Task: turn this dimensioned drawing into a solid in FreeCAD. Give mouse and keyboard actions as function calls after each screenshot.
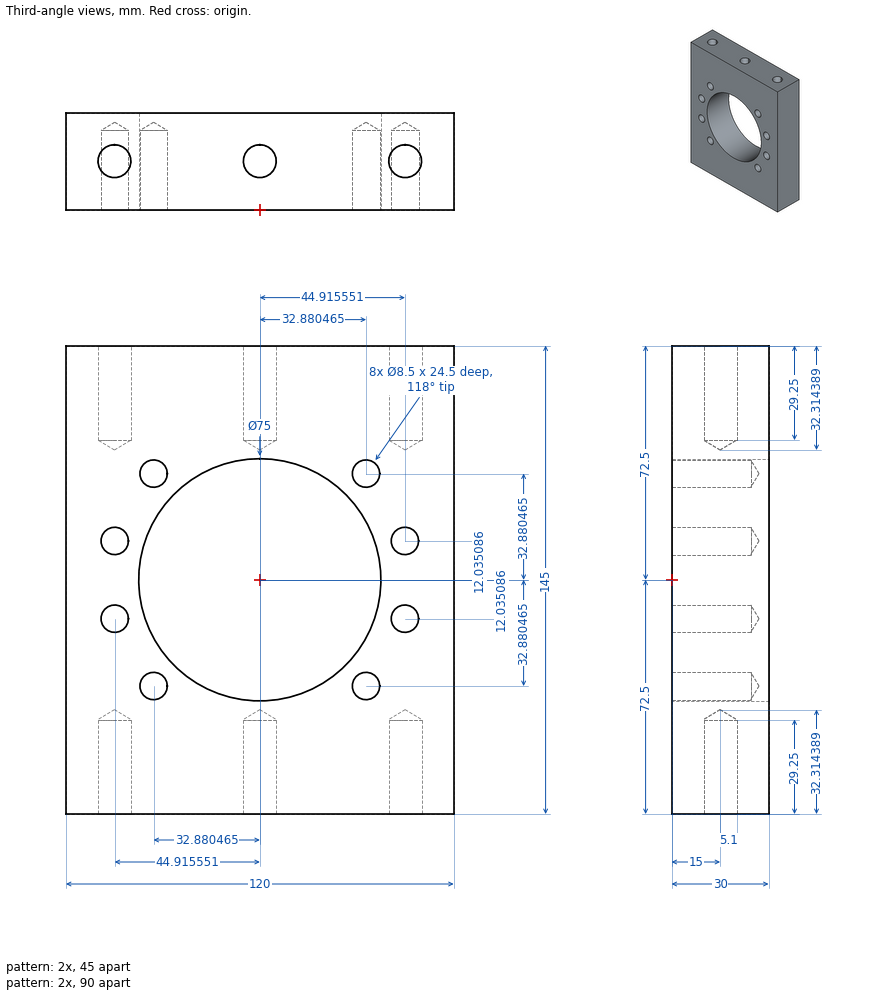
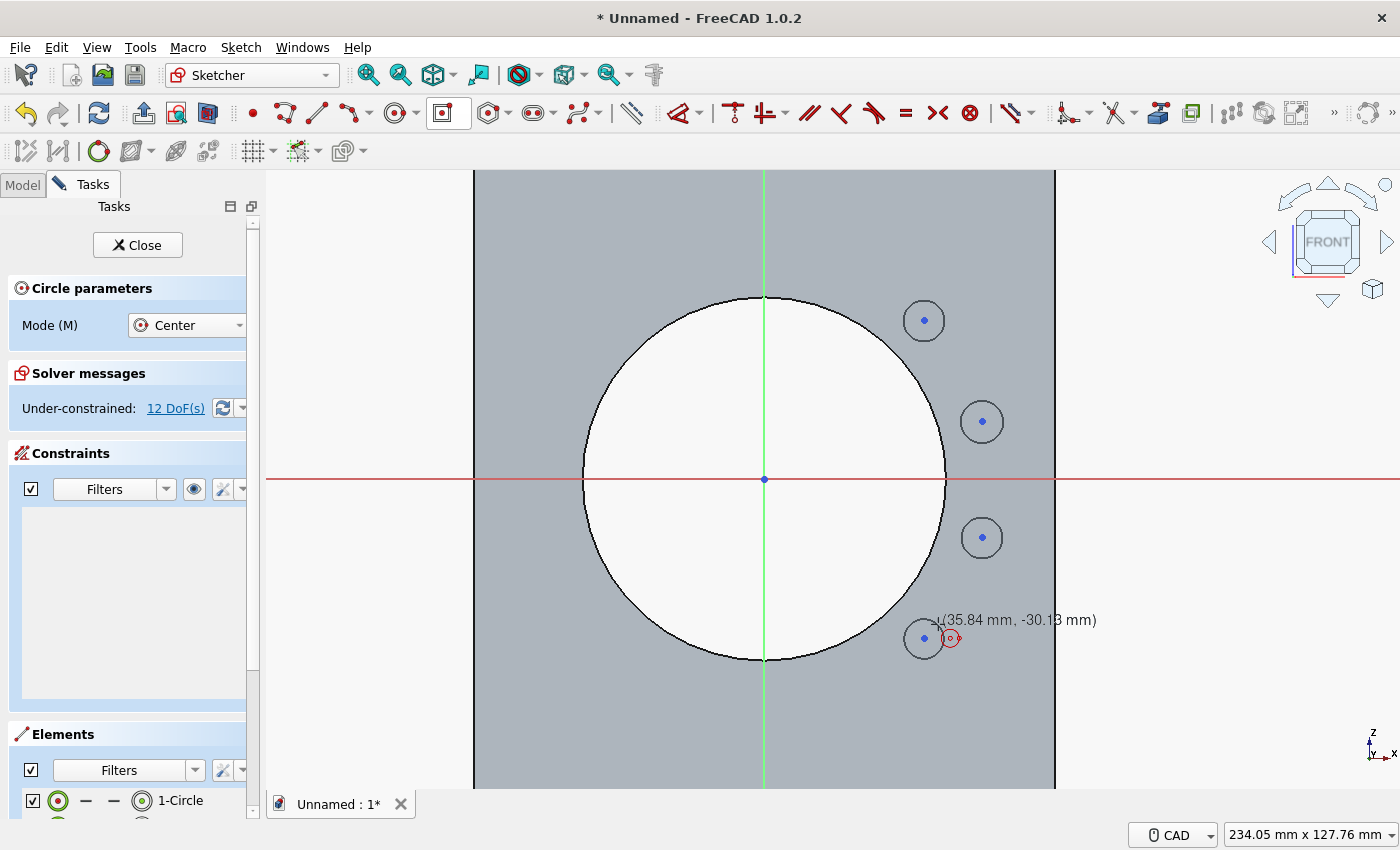
click(605, 638)
click(620, 624)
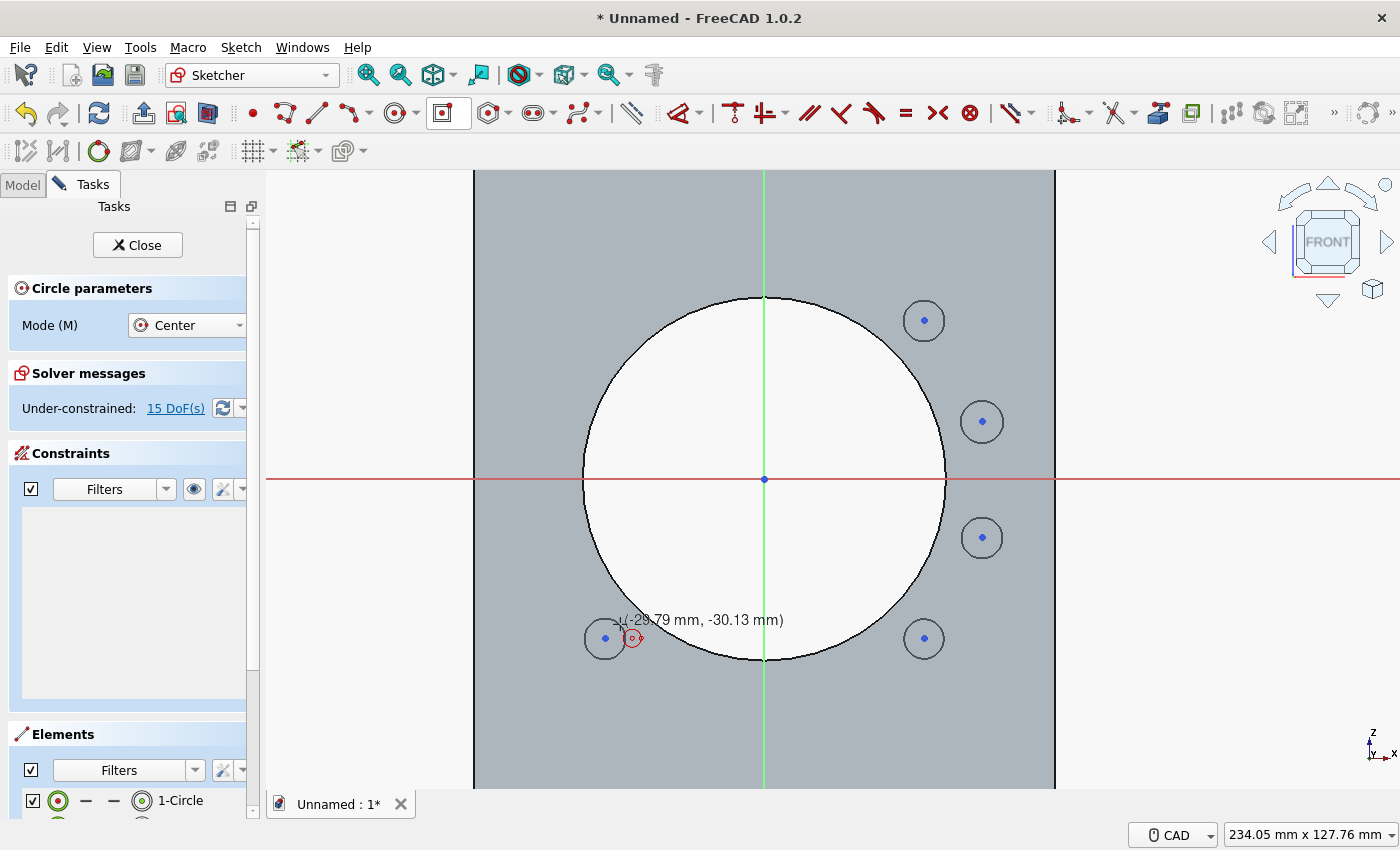
click(547, 537)
click(561, 523)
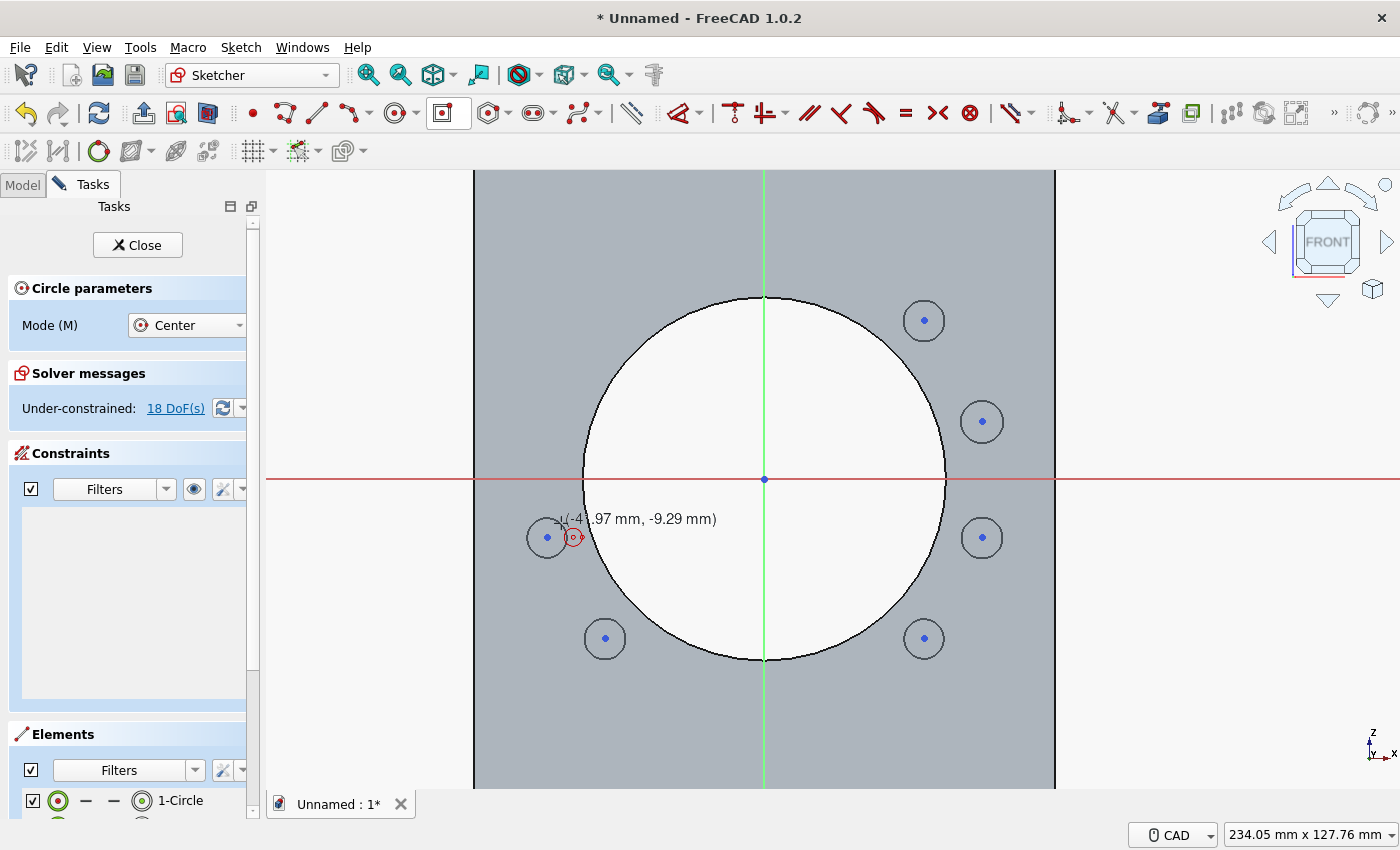
click(547, 421)
click(561, 406)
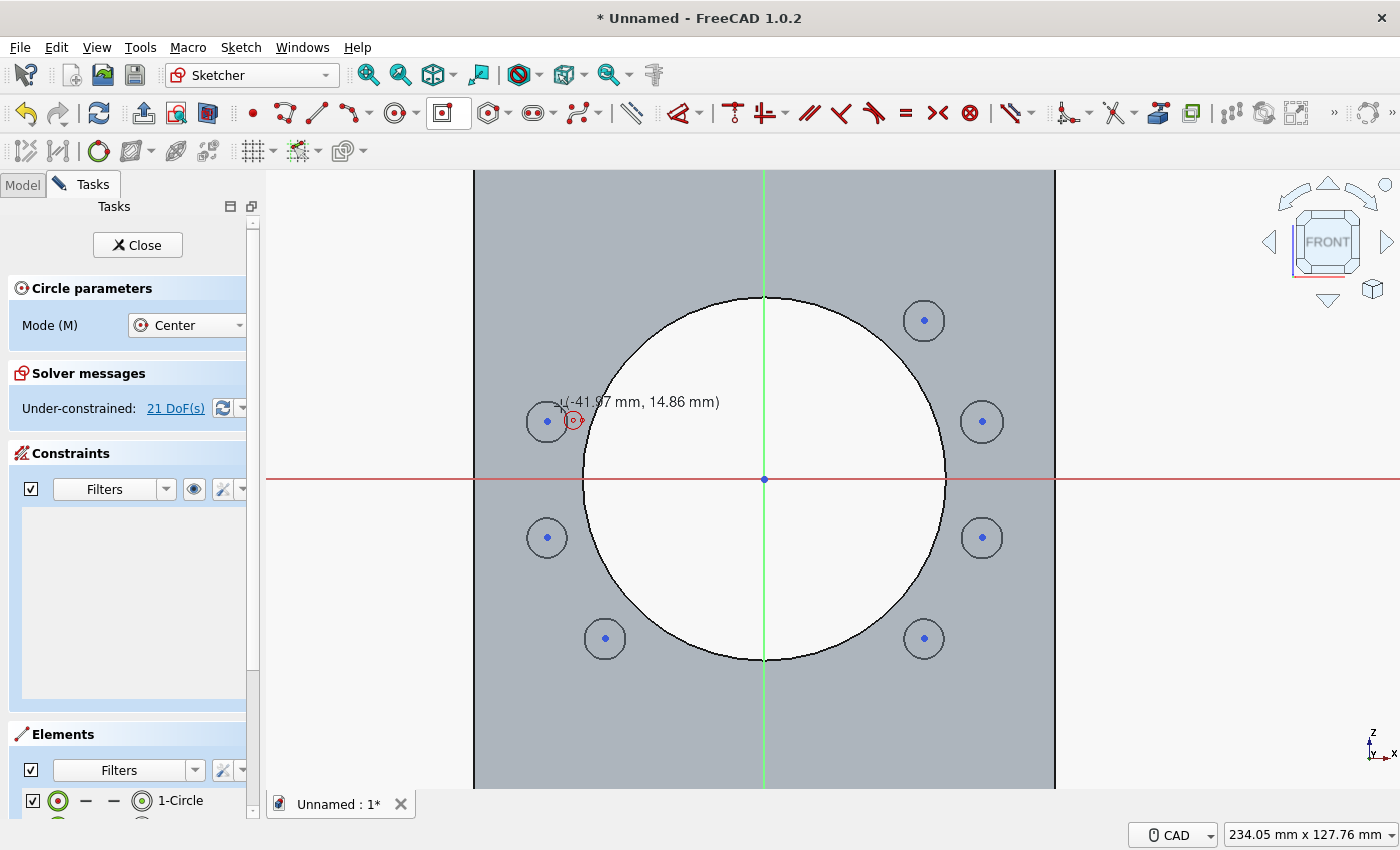
click(605, 320)
click(620, 305)
key(Escape)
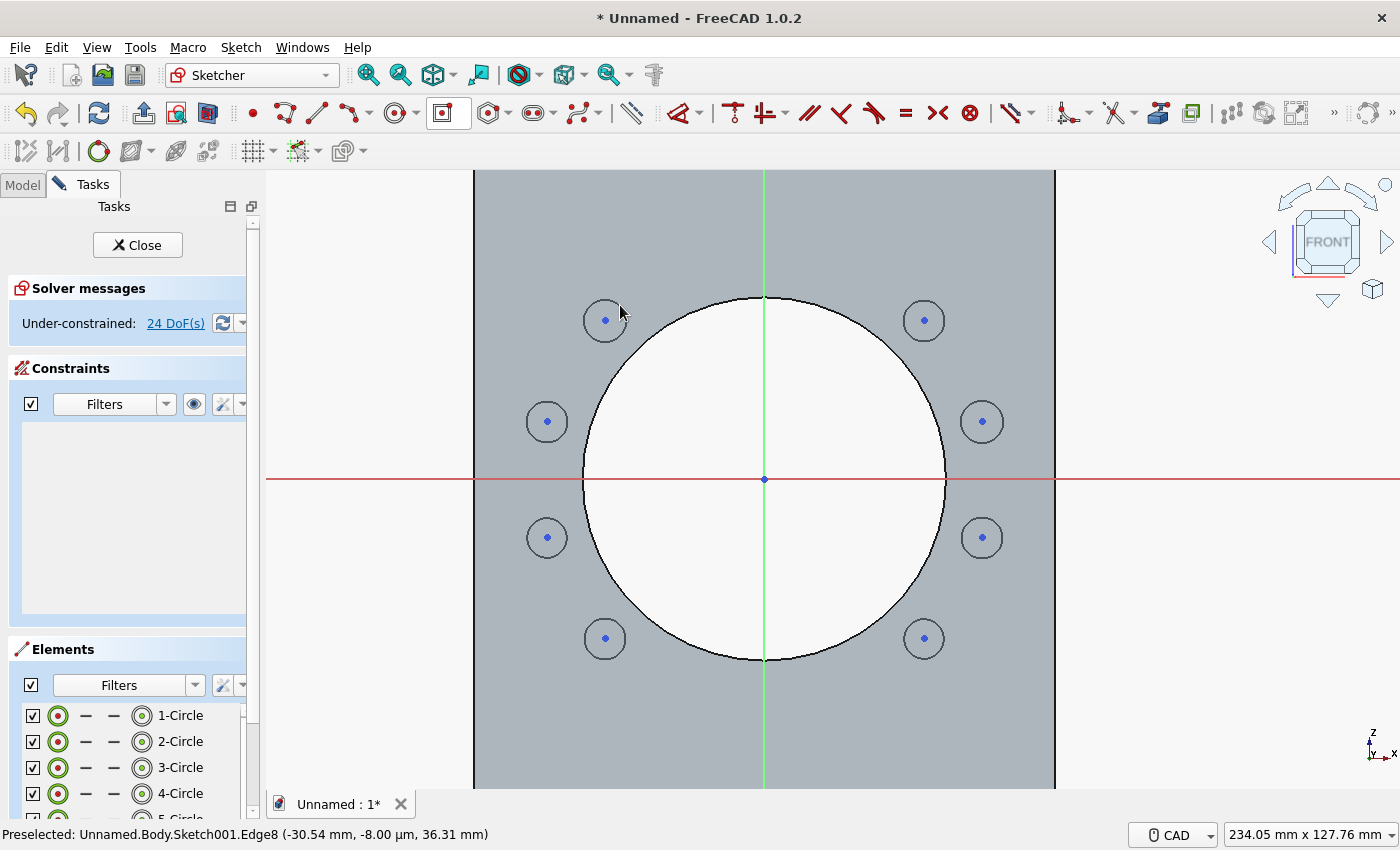
click(938, 306)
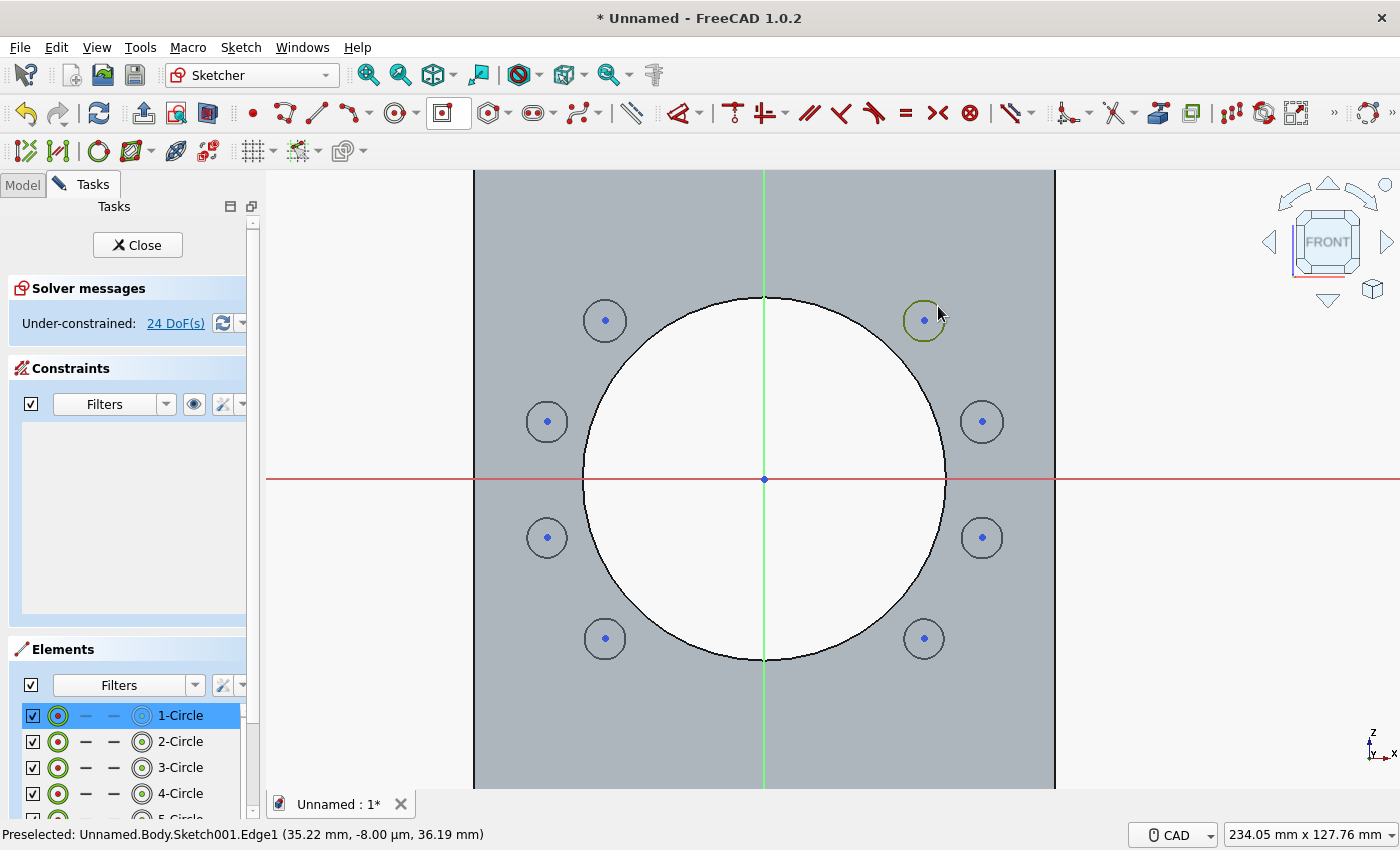
click(997, 407)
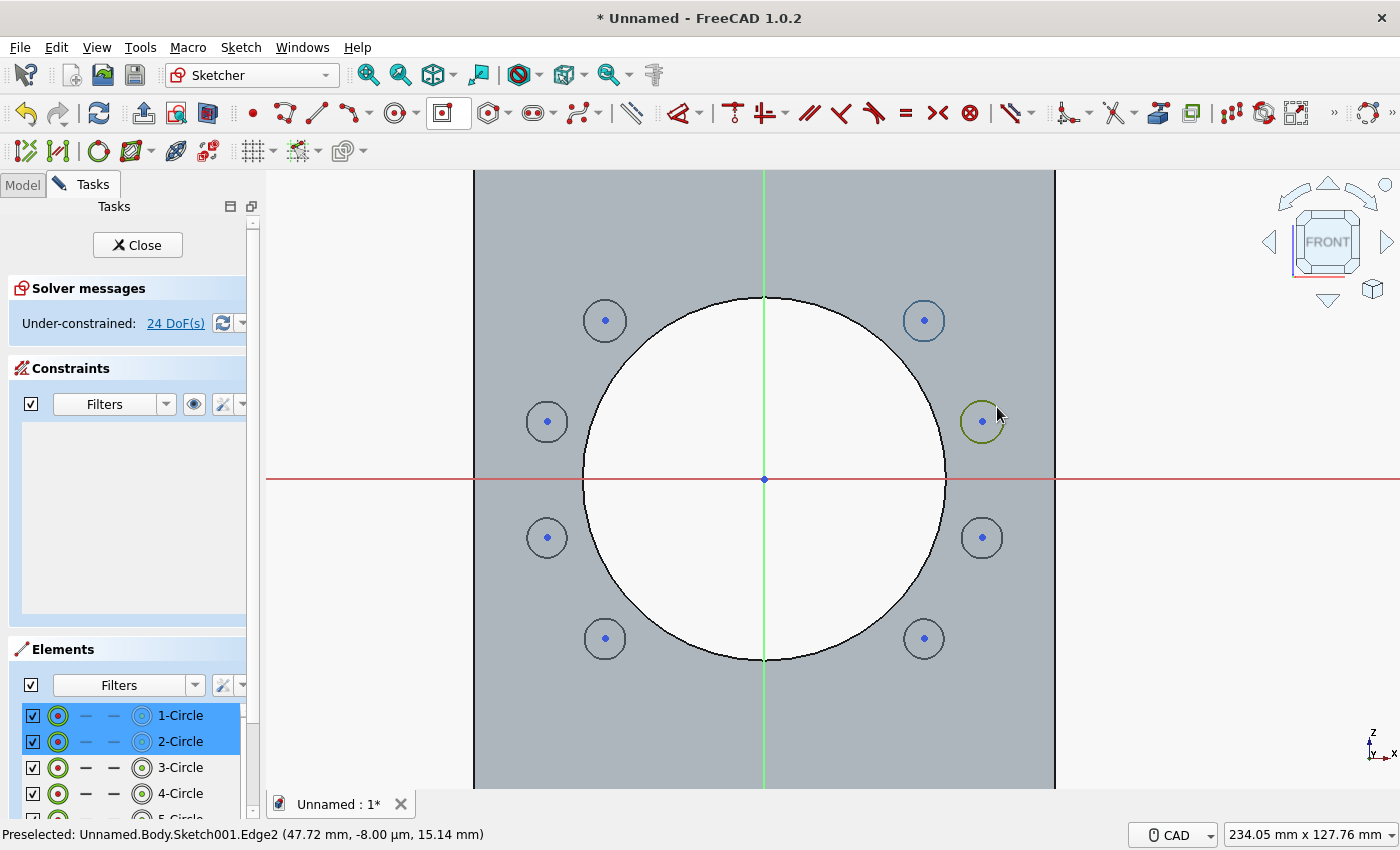
click(996, 523)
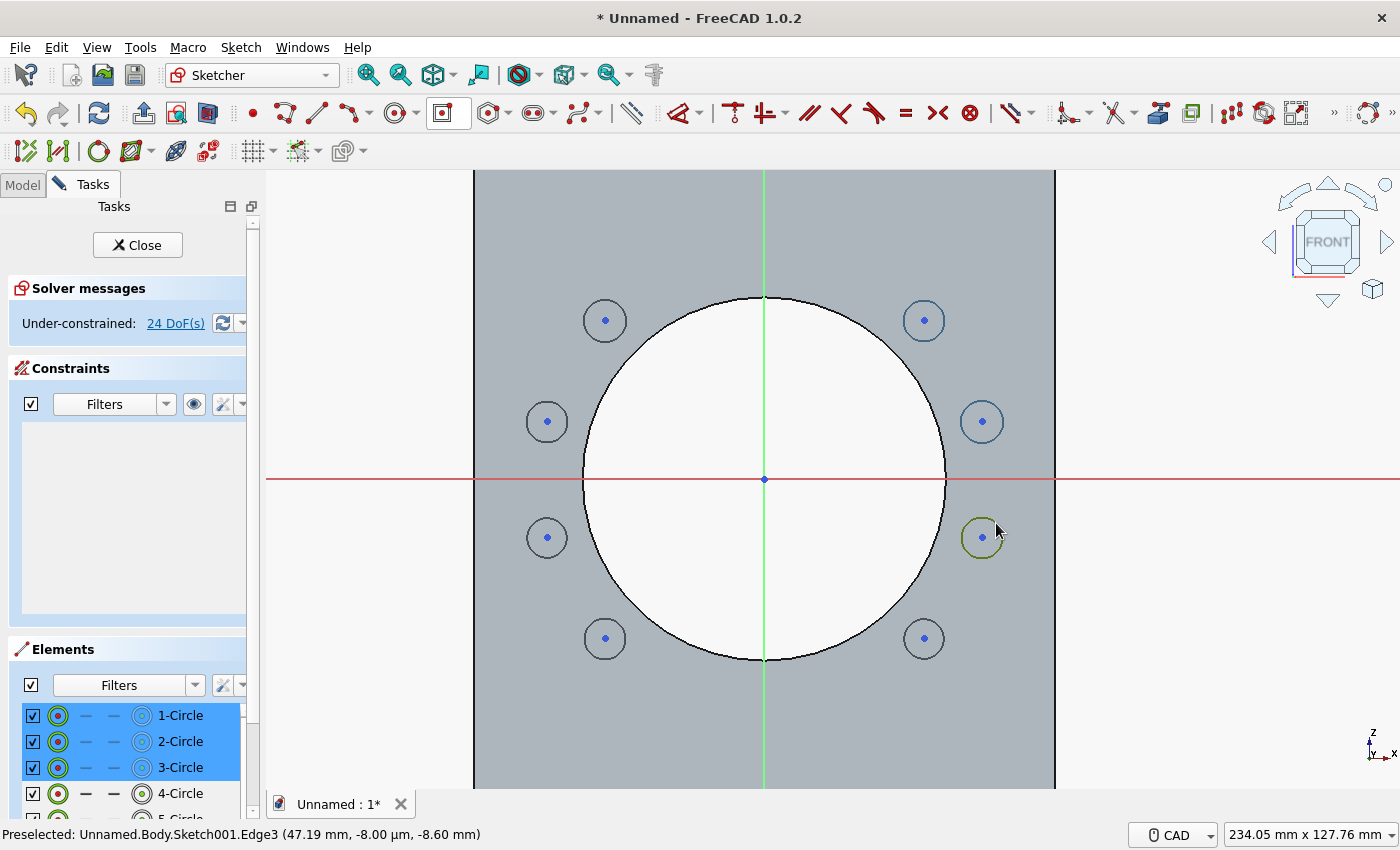
click(938, 625)